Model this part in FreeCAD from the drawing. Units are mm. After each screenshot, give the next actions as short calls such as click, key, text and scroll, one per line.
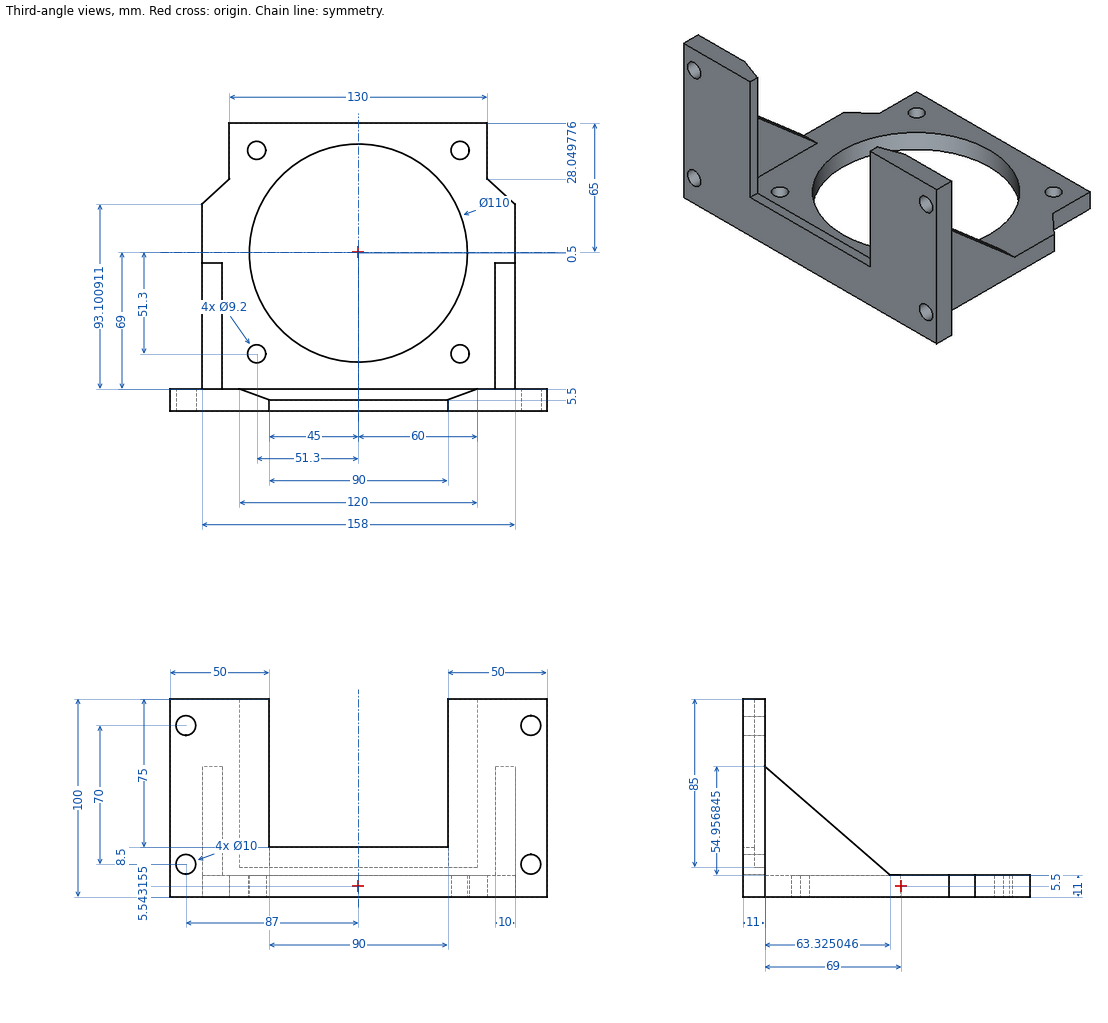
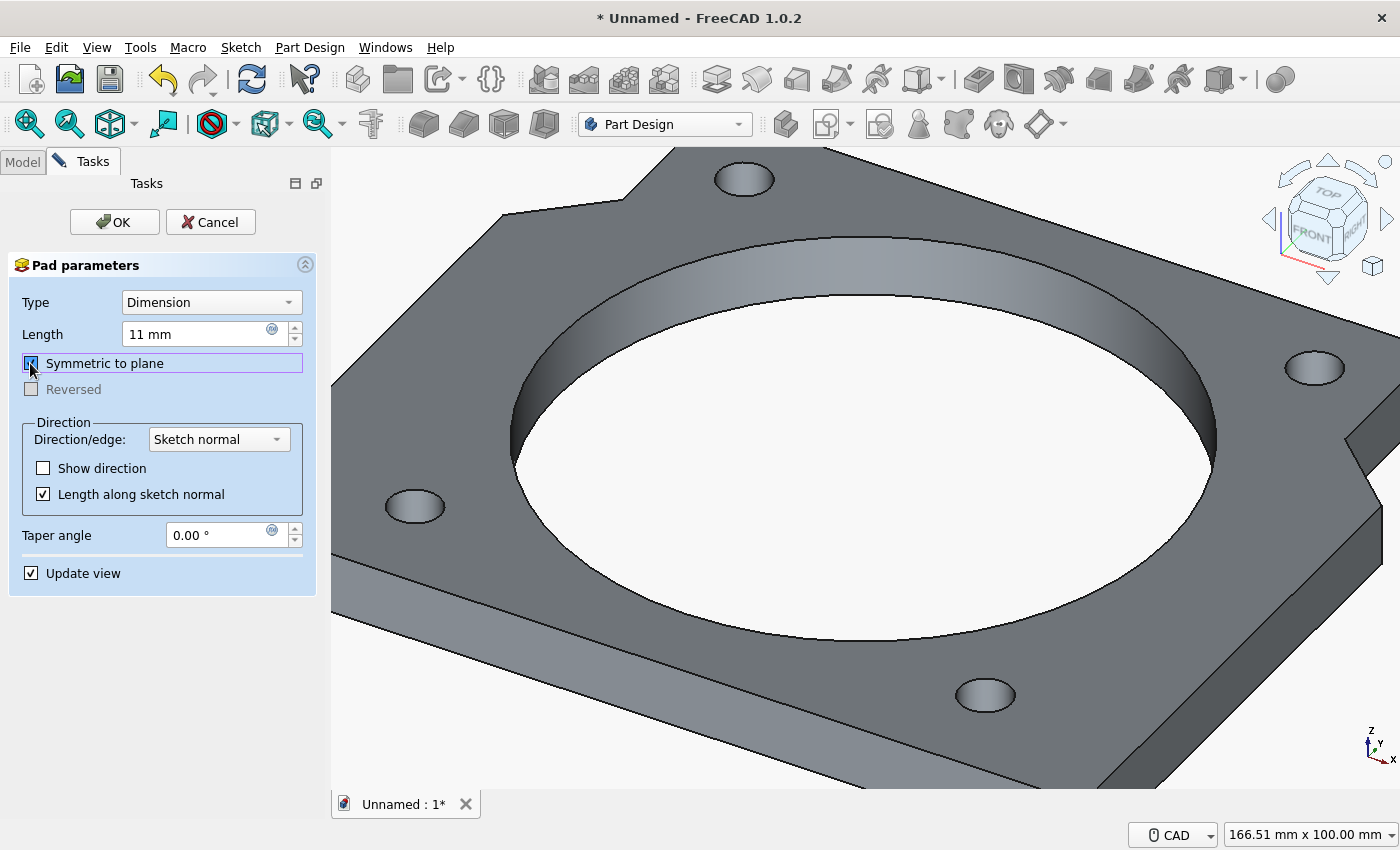
click(115, 222)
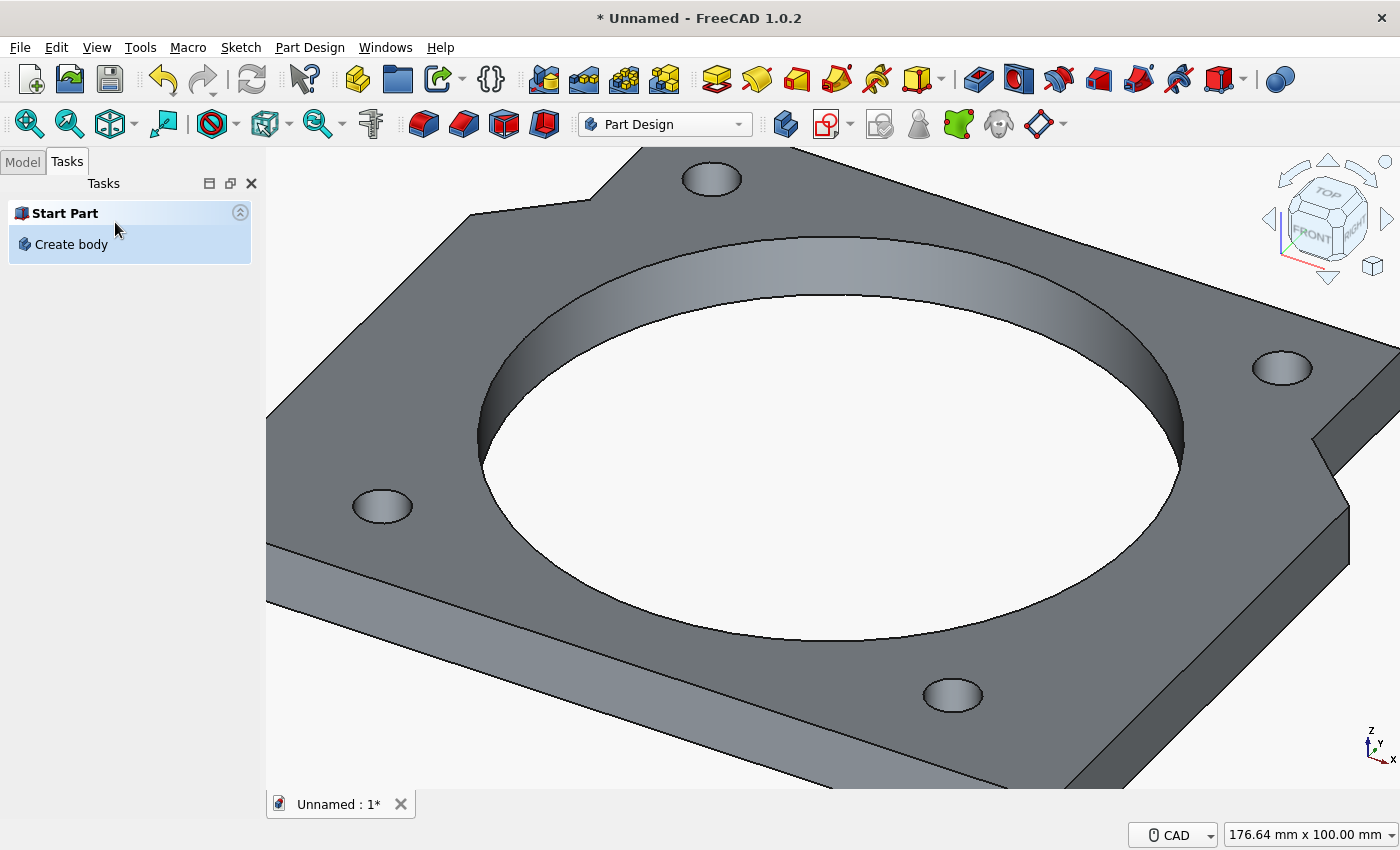
click(30, 124)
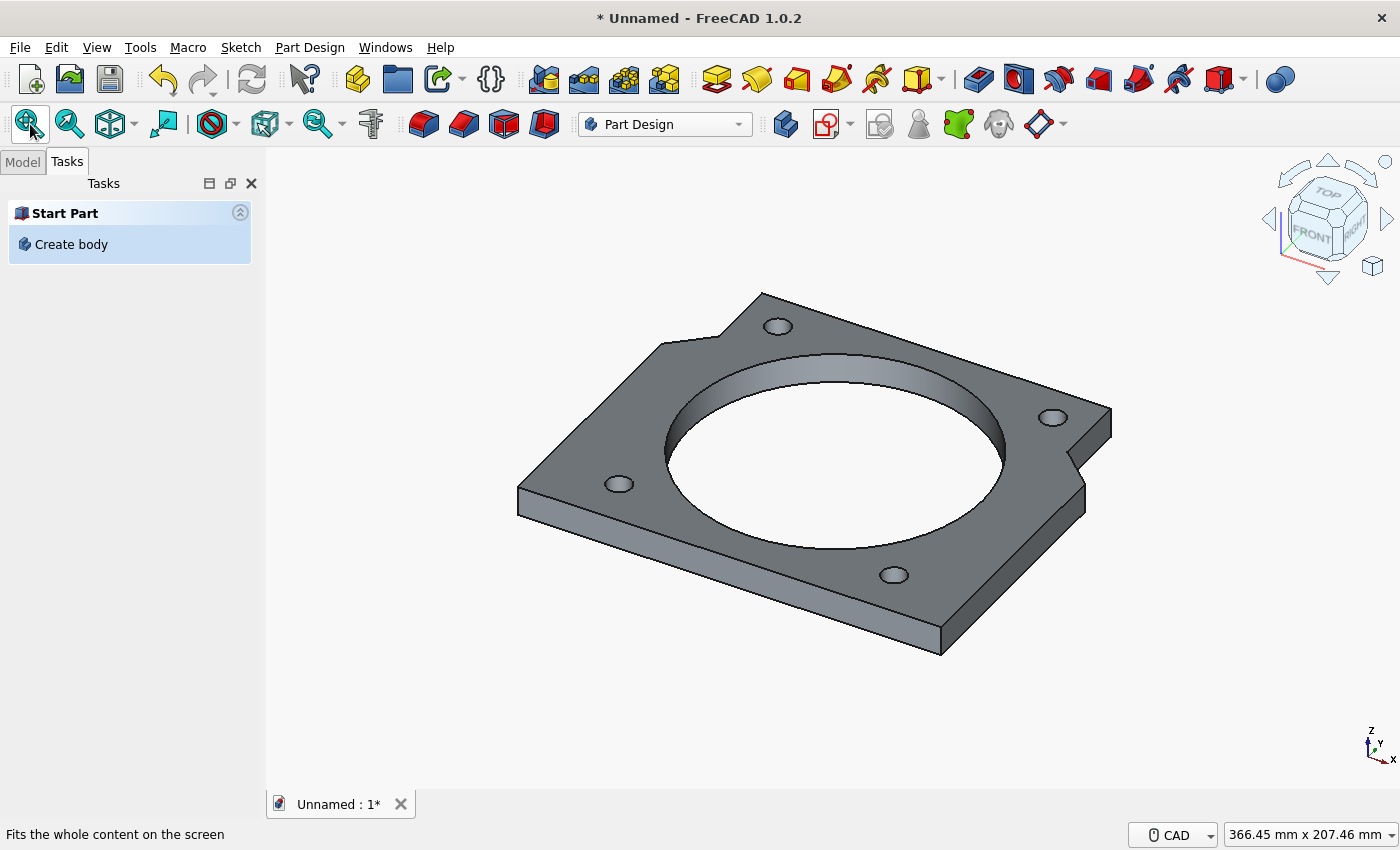
click(911, 630)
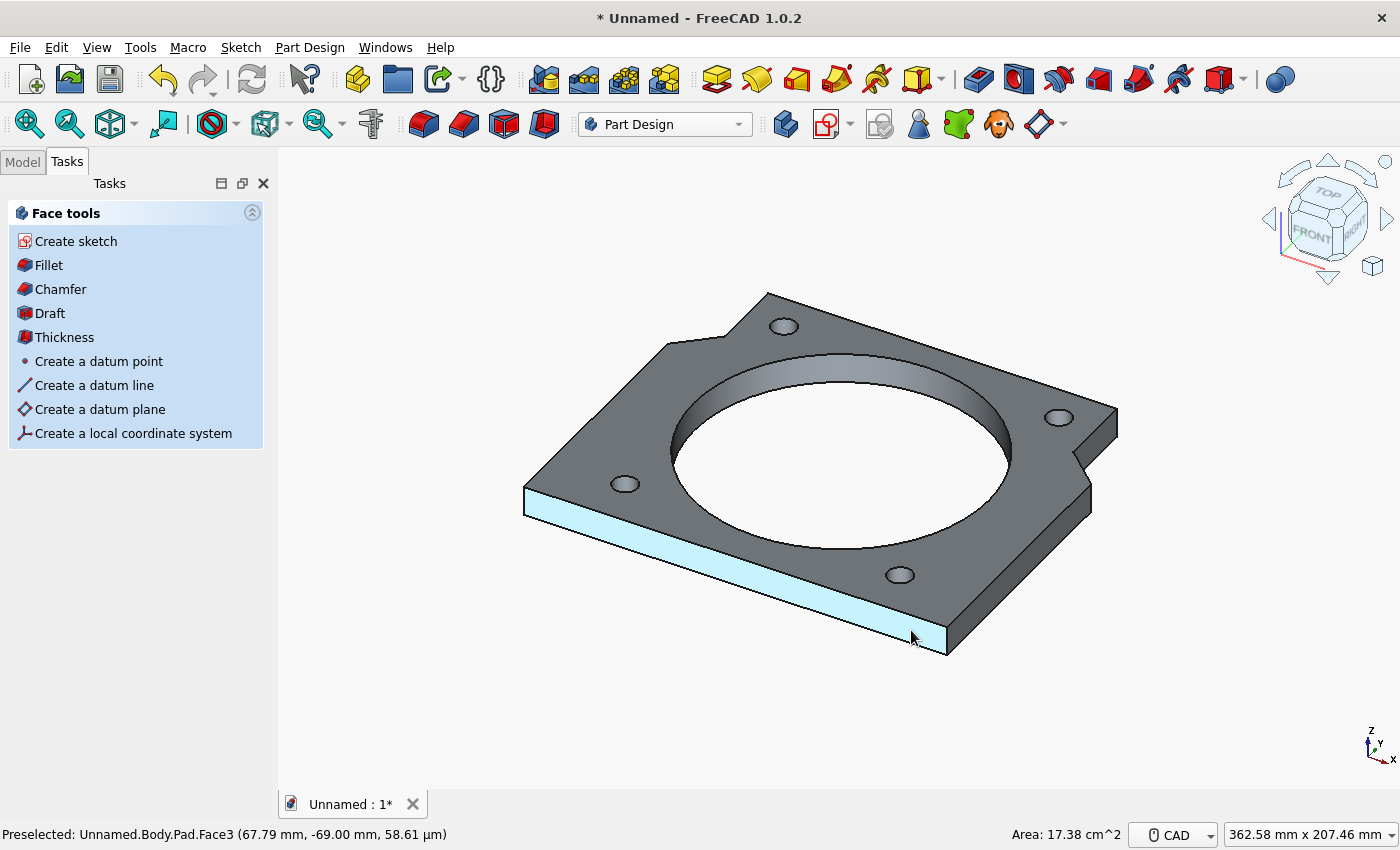
click(826, 124)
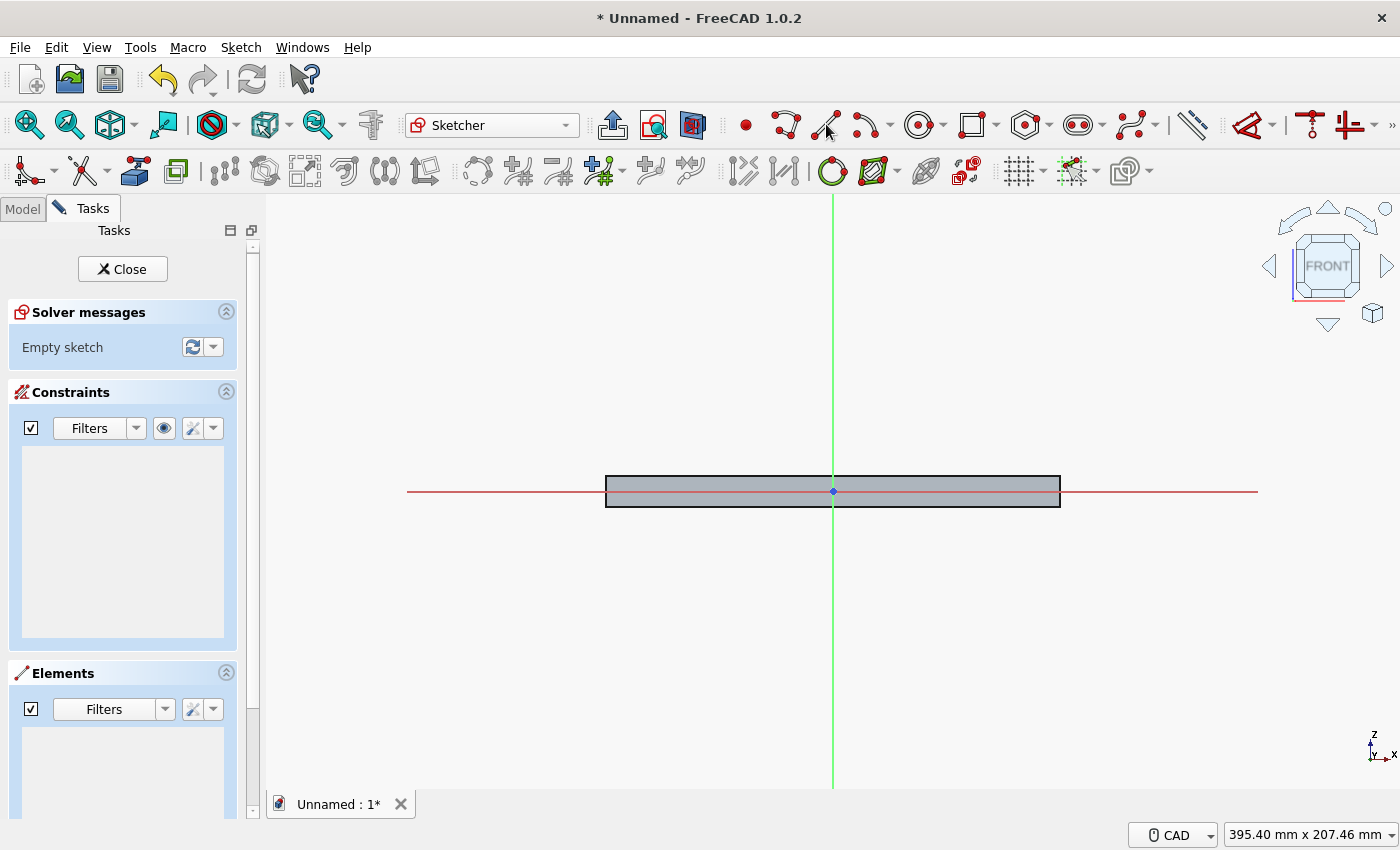
scroll(455, 761, down, 1)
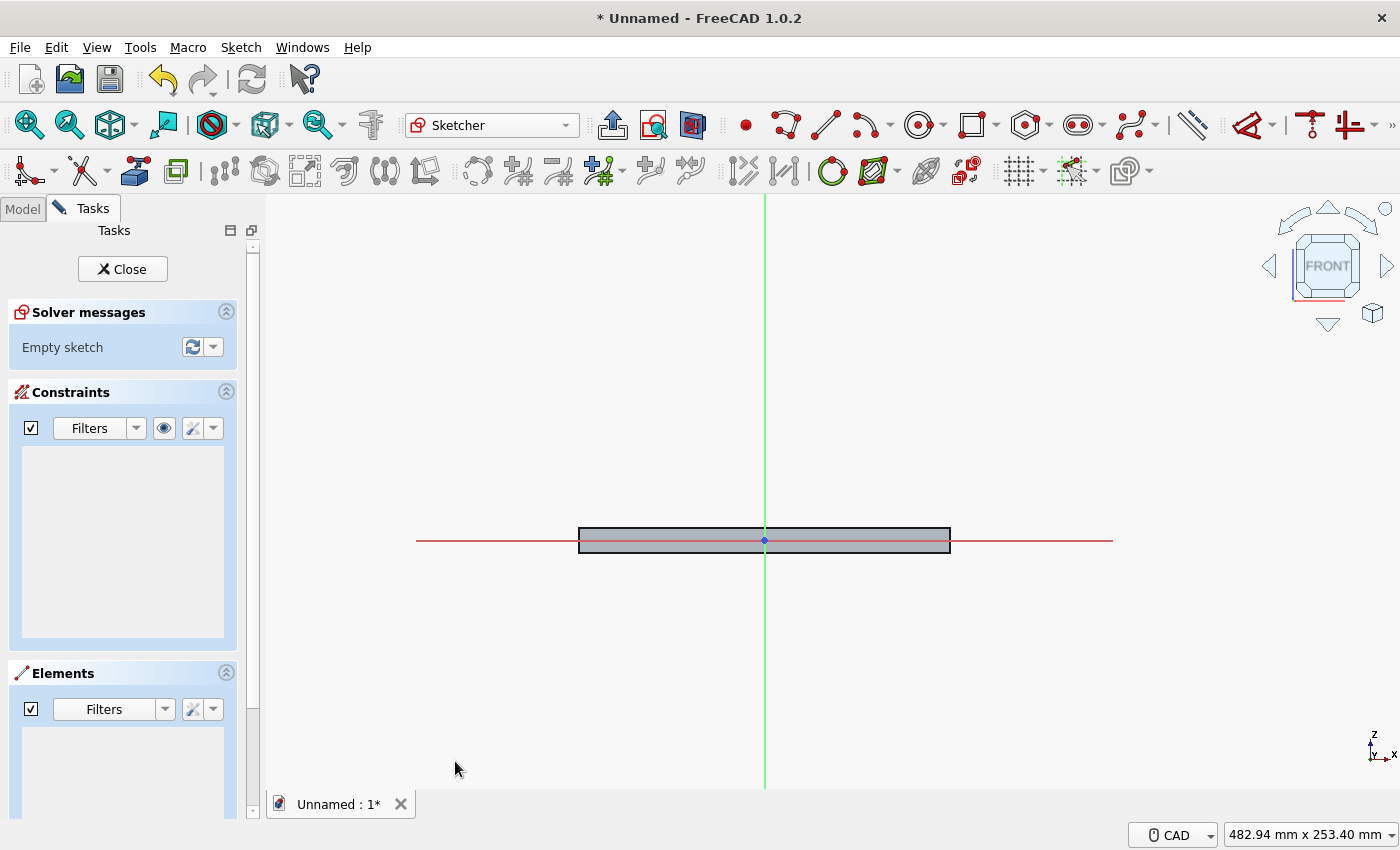
scroll(765, 324, up, 2)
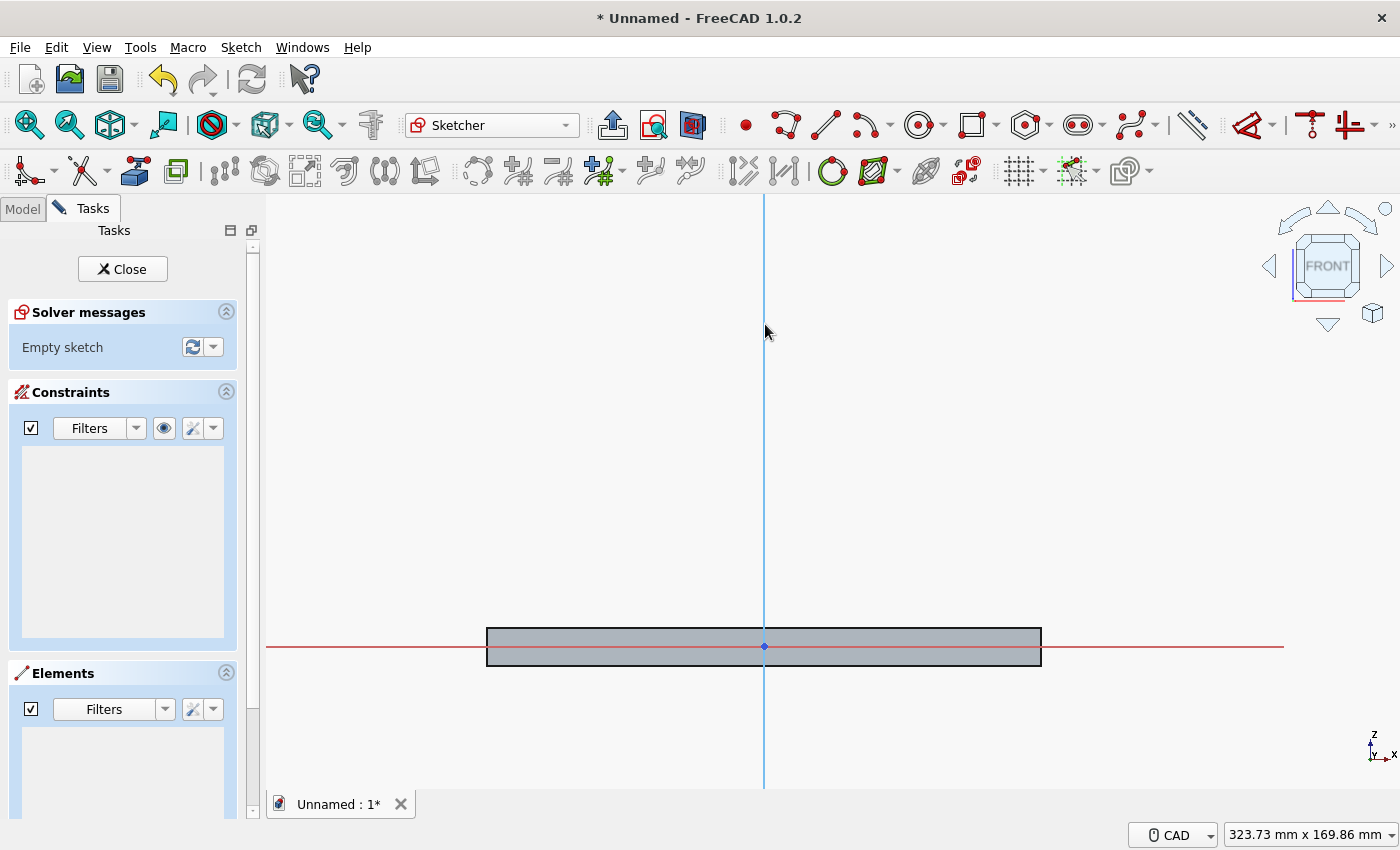
key(g)
key(m)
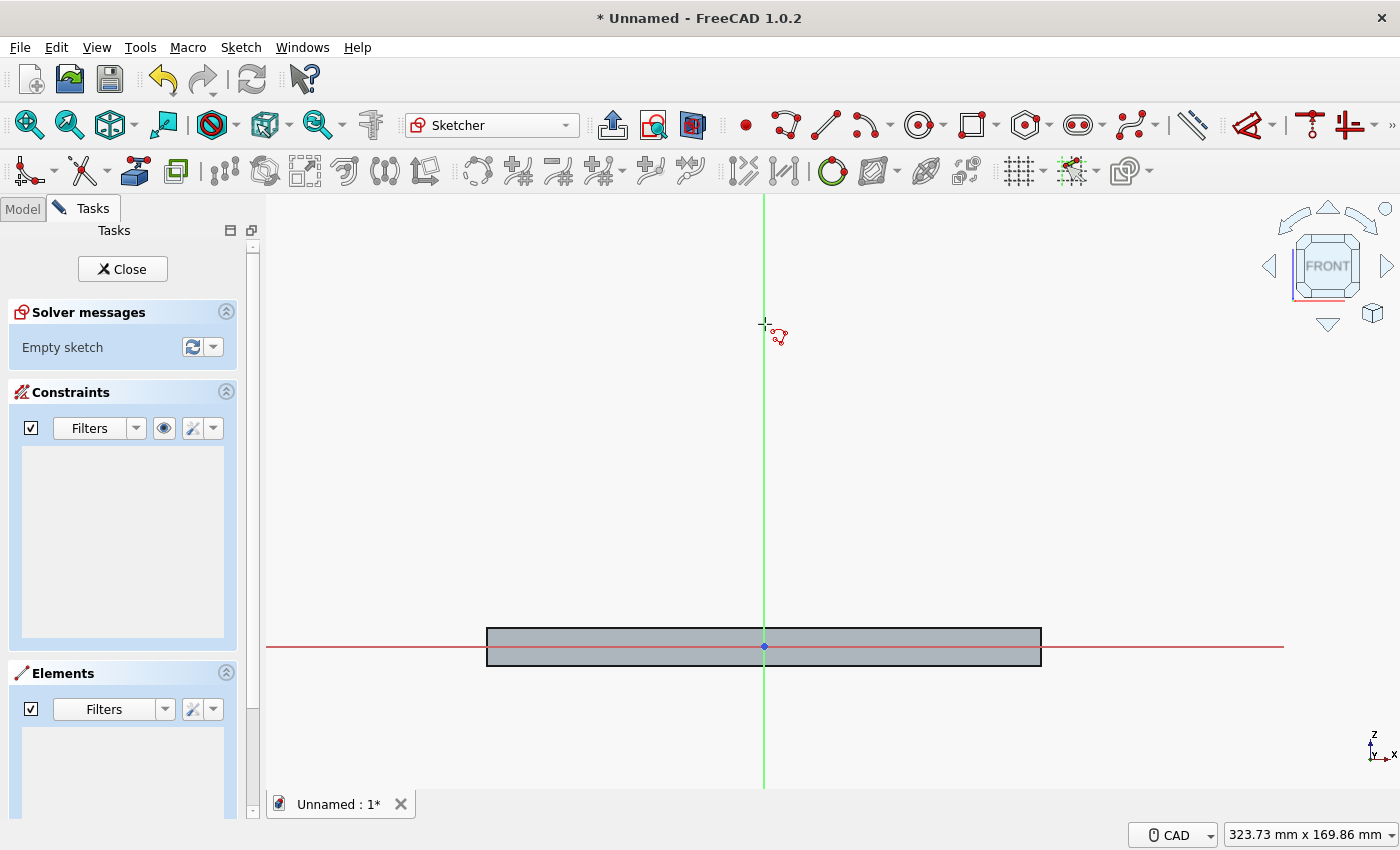
click(922, 579)
click(606, 579)
click(606, 316)
click(431, 316)
click(431, 666)
click(1097, 666)
click(1097, 316)
click(922, 316)
click(922, 580)